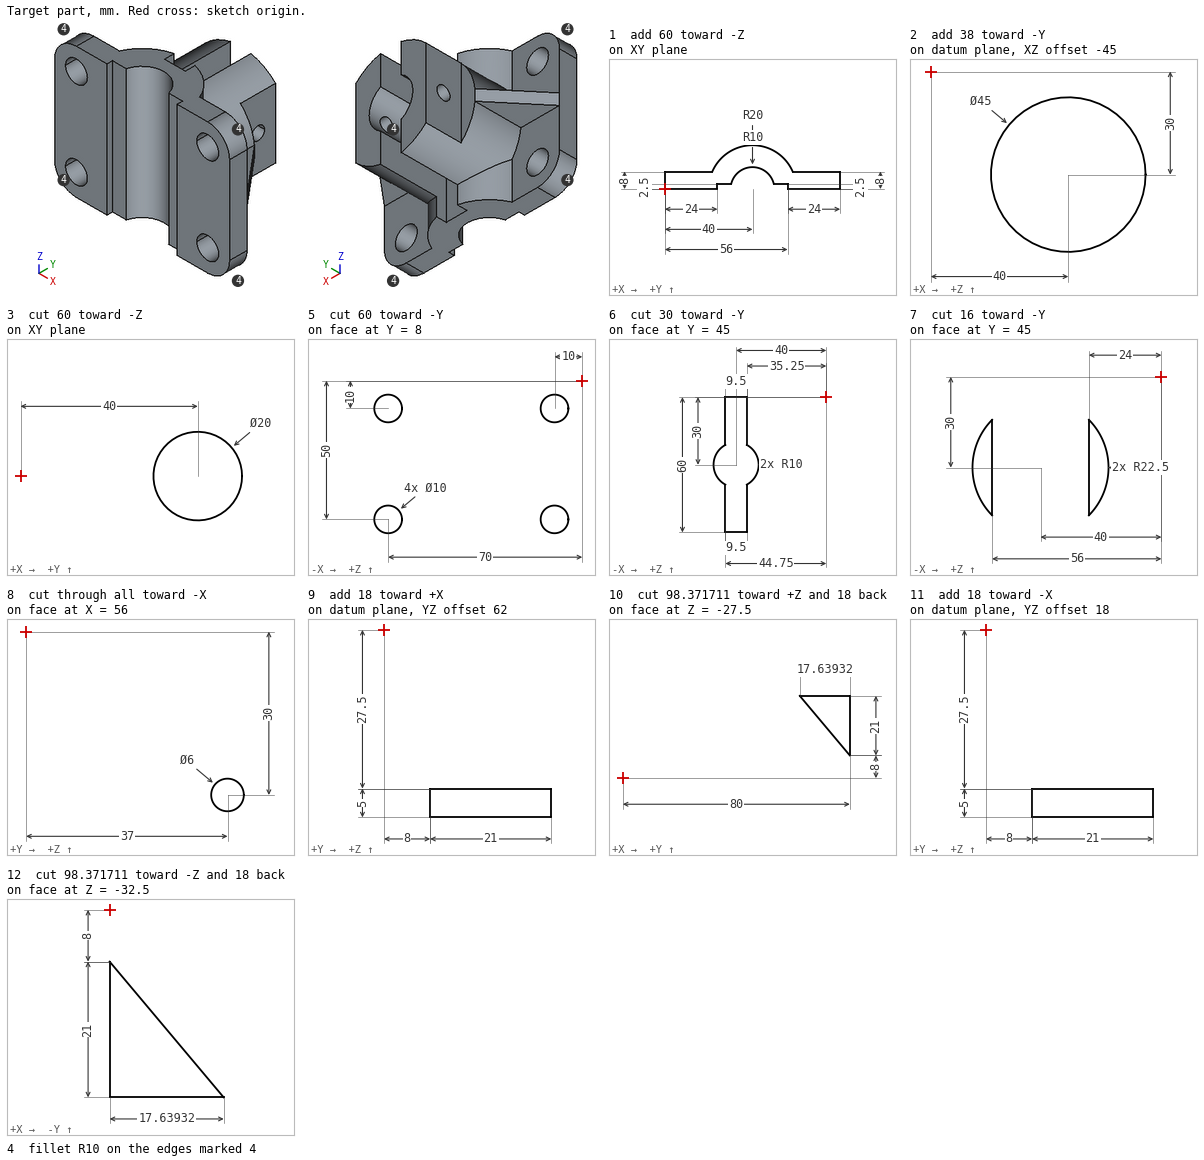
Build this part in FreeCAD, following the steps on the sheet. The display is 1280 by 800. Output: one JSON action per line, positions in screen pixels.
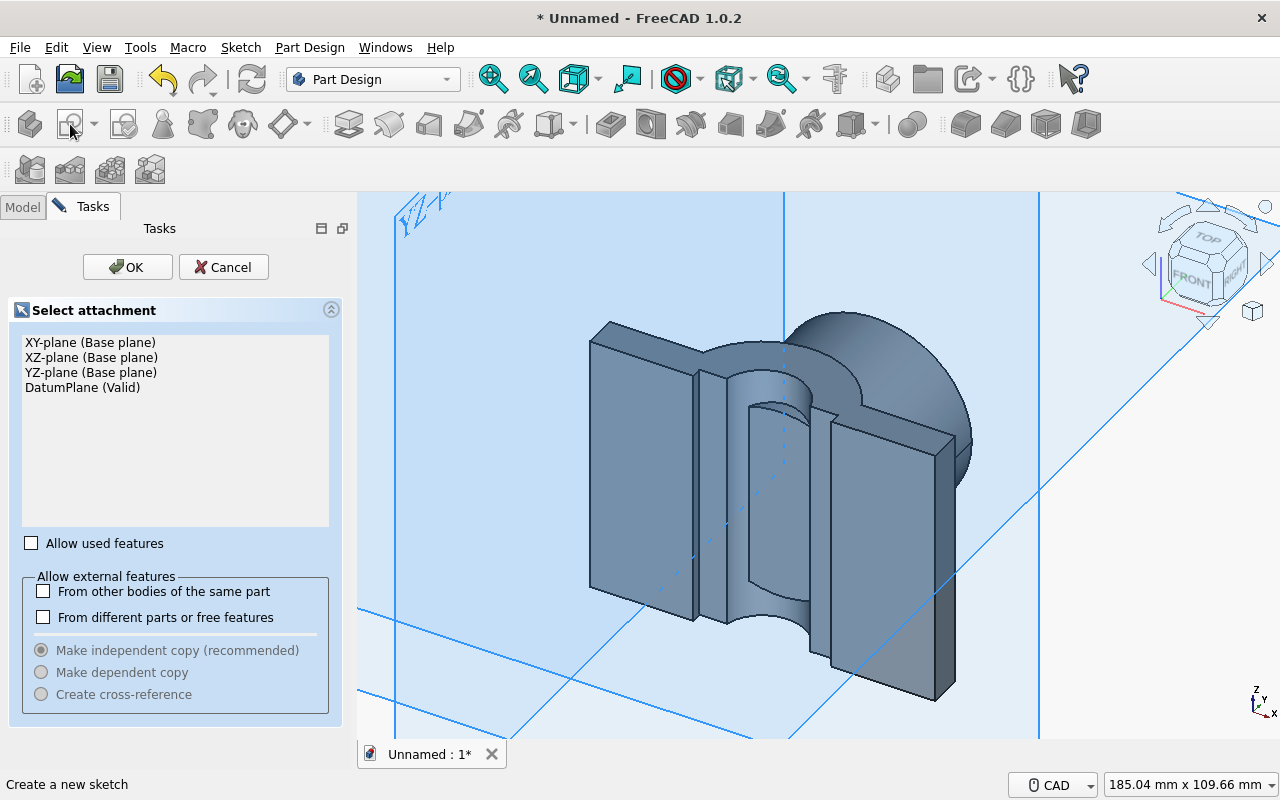
{"action": "left_click", "coordinate": [82, 342]}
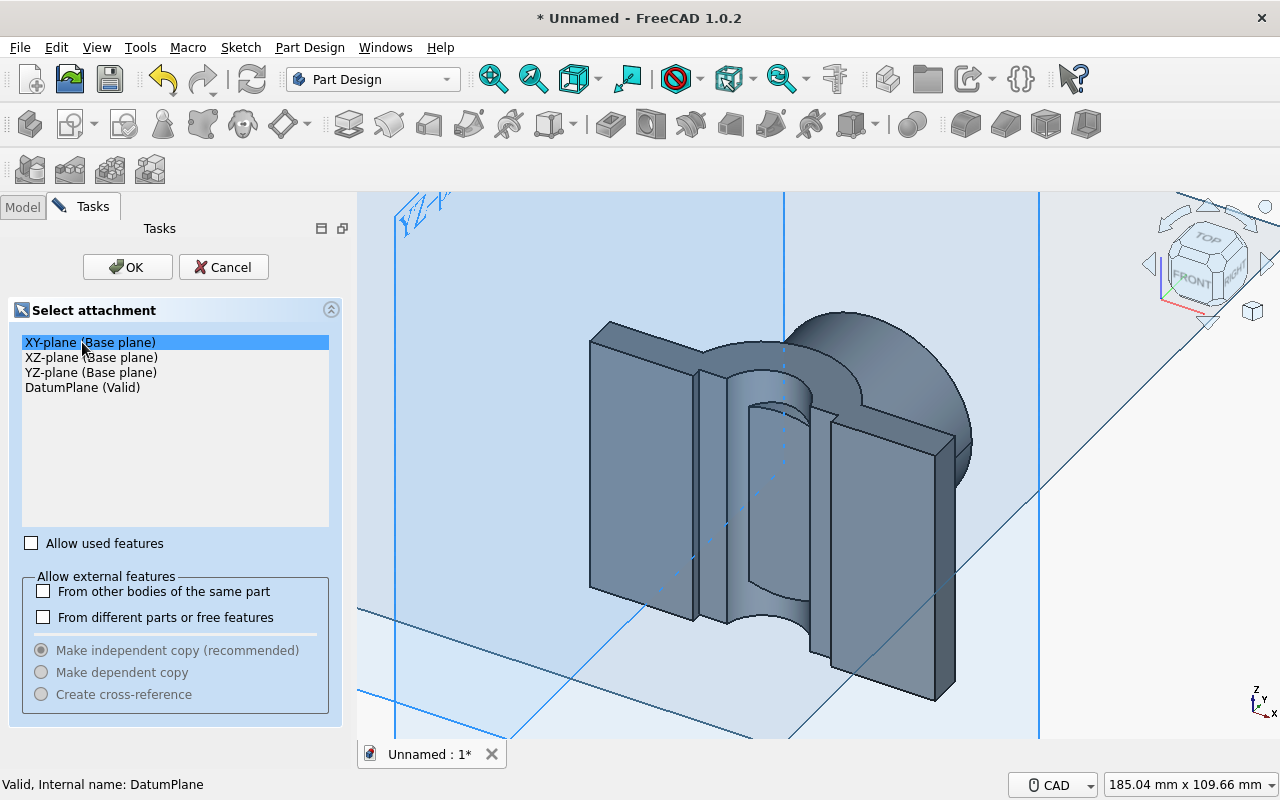
{"action": "left_click", "coordinate": [128, 267]}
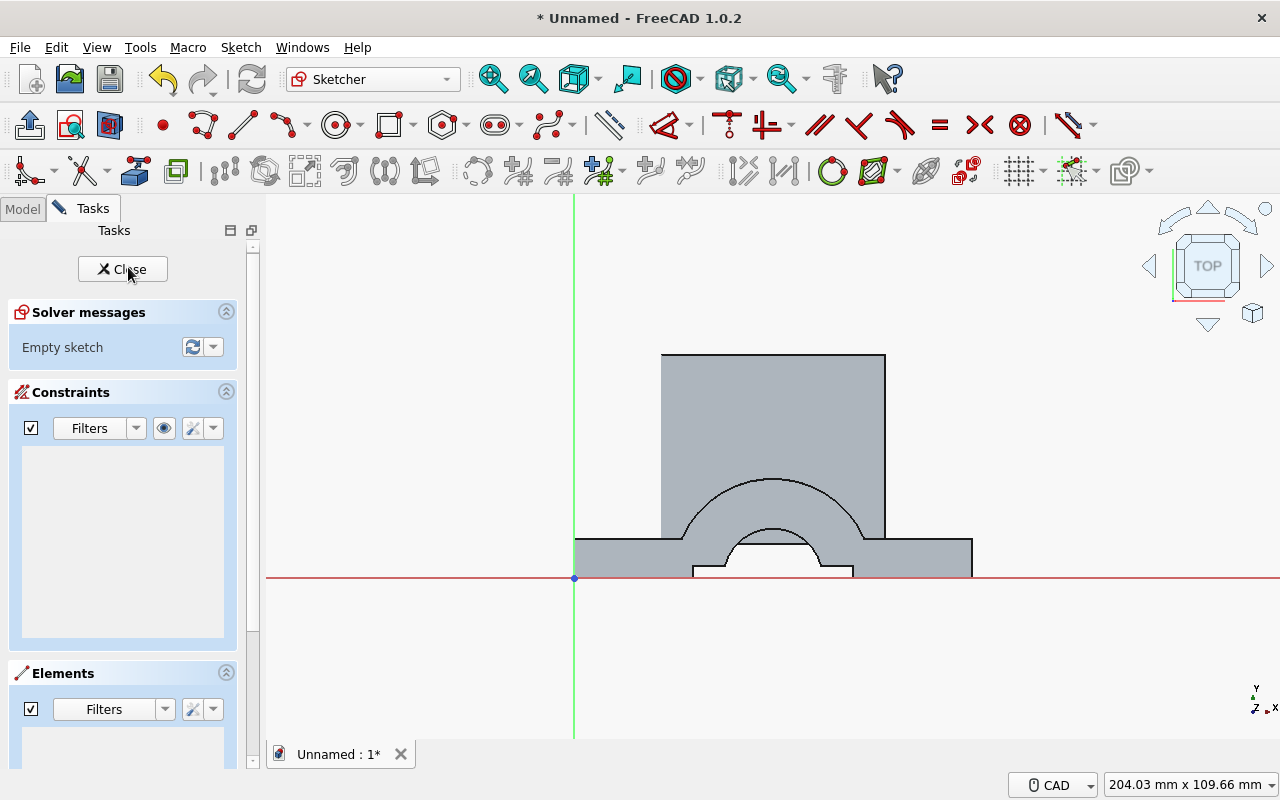
{"action": "scroll", "coordinate": [803, 627], "scroll_direction": "up", "scroll_amount": 6}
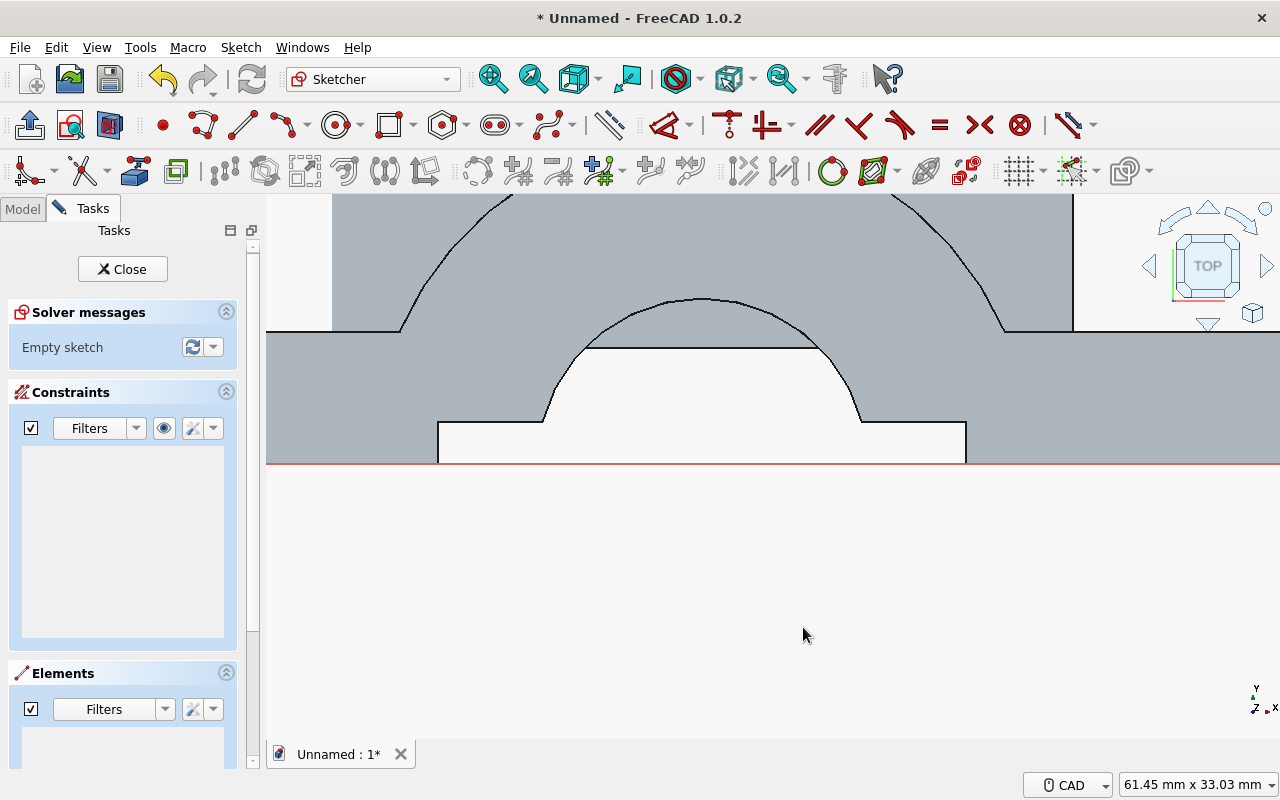
{"action": "left_click", "coordinate": [336, 126]}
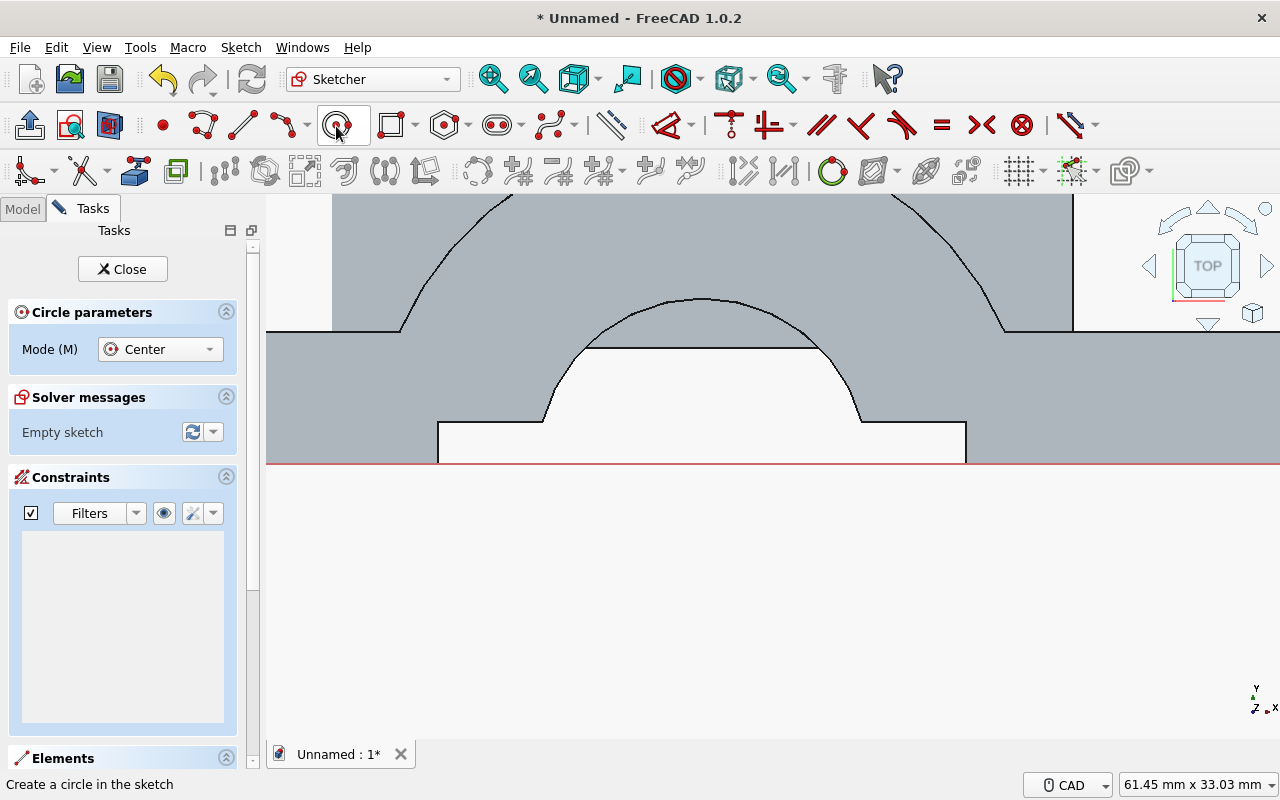
{"action": "left_click", "coordinate": [702, 464]}
{"action": "left_click", "coordinate": [819, 347]}
{"action": "key", "text": "Escape"}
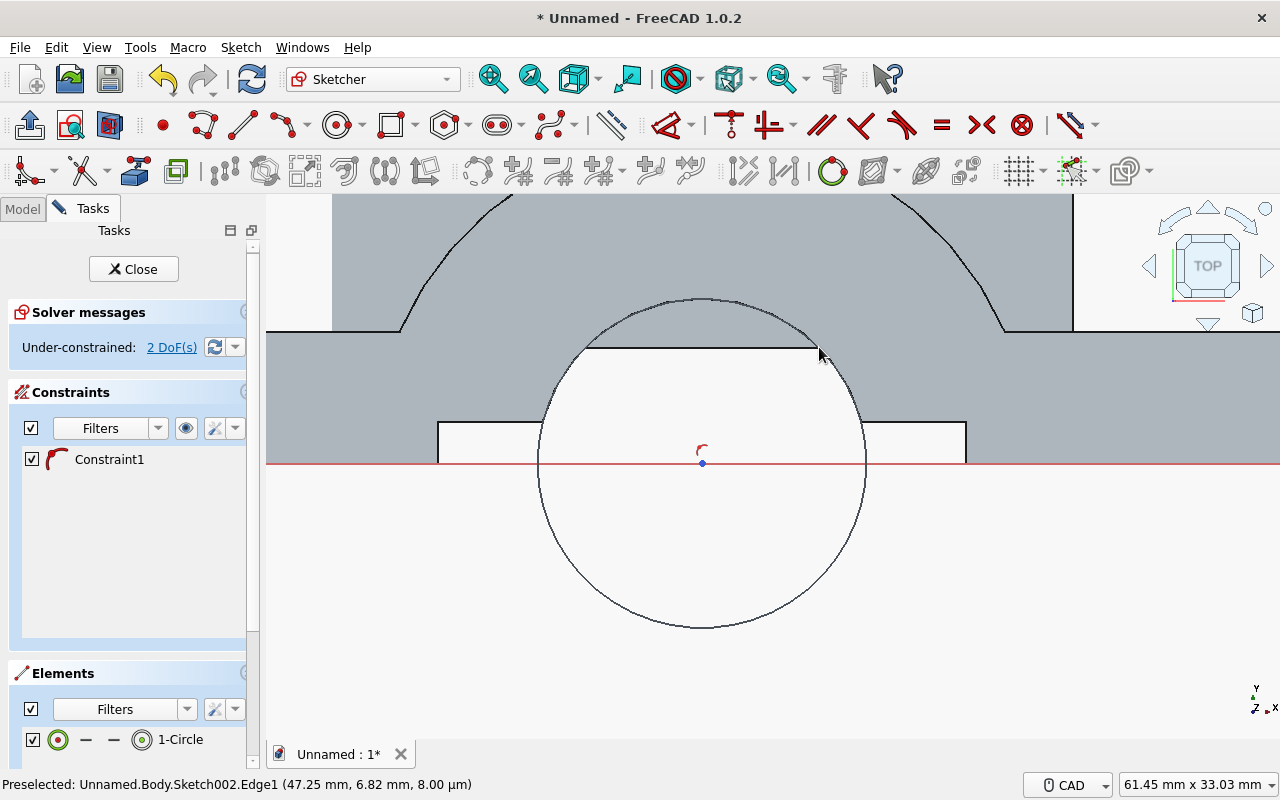
{"action": "left_click", "coordinate": [666, 126]}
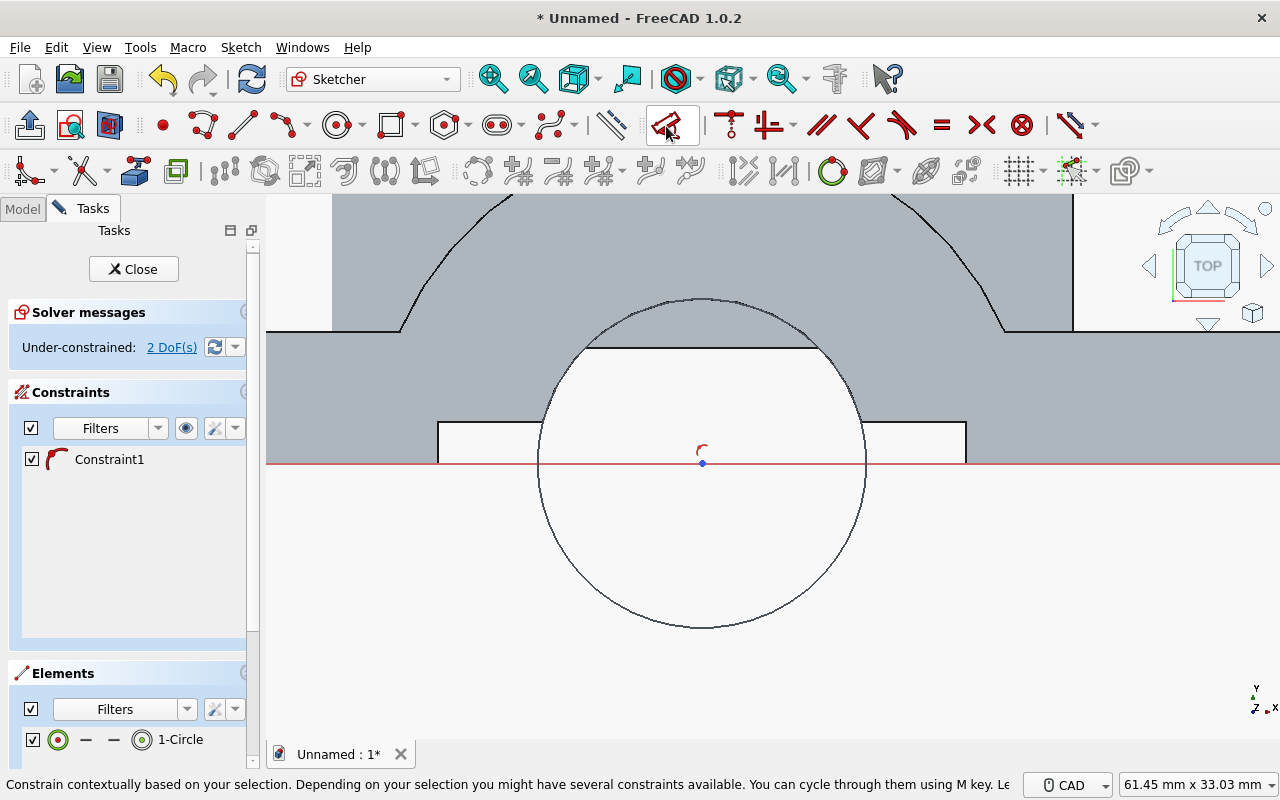
{"action": "left_click", "coordinate": [818, 347]}
{"action": "left_click", "coordinate": [841, 324]}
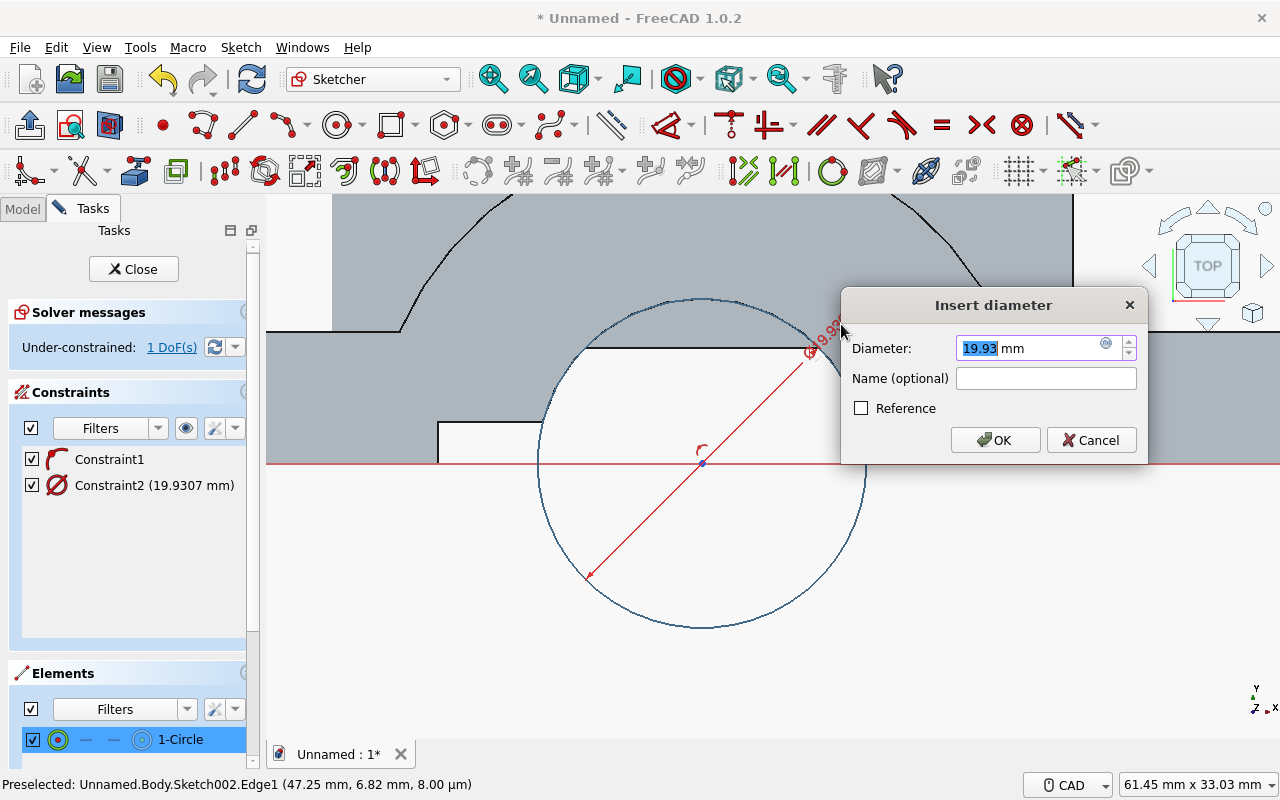
{"action": "type", "text": "20"}
{"action": "key", "text": "Return"}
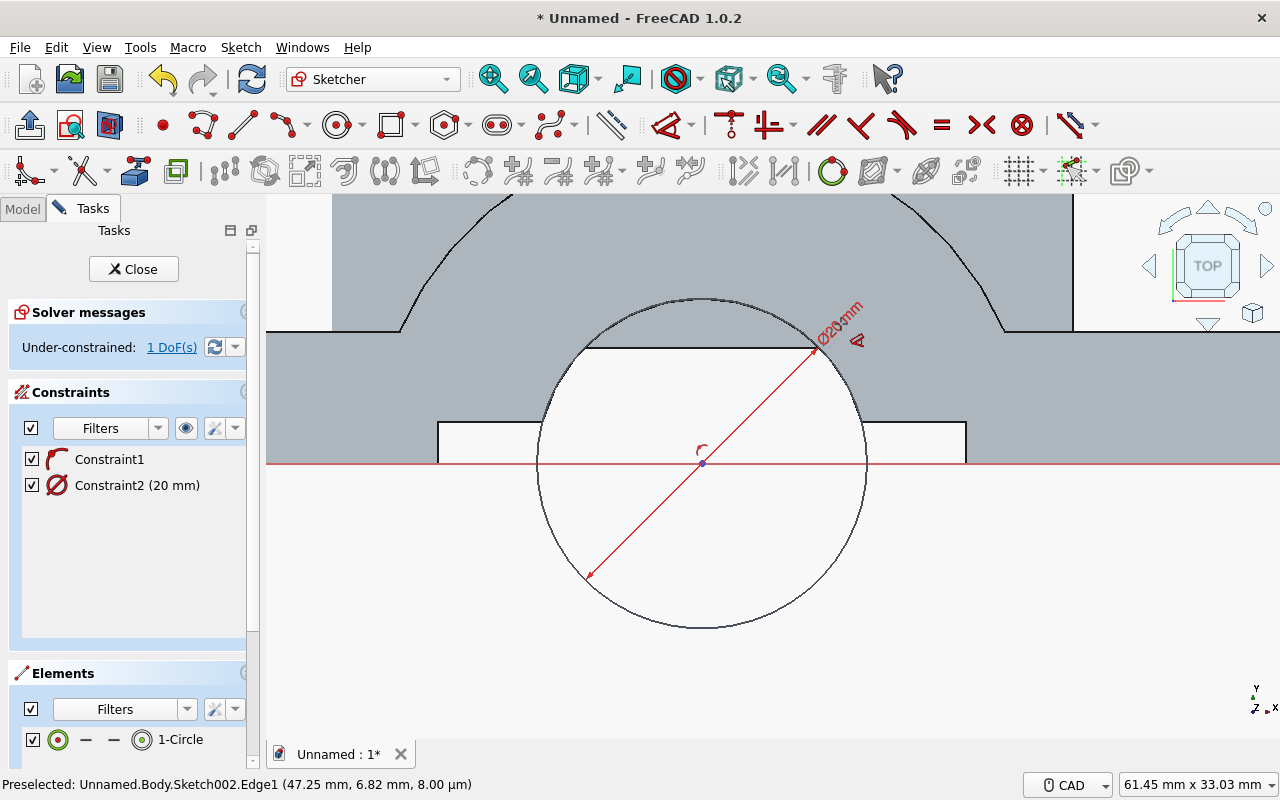
{"action": "left_click", "coordinate": [702, 464]}
{"action": "left_click", "coordinate": [498, 498]}